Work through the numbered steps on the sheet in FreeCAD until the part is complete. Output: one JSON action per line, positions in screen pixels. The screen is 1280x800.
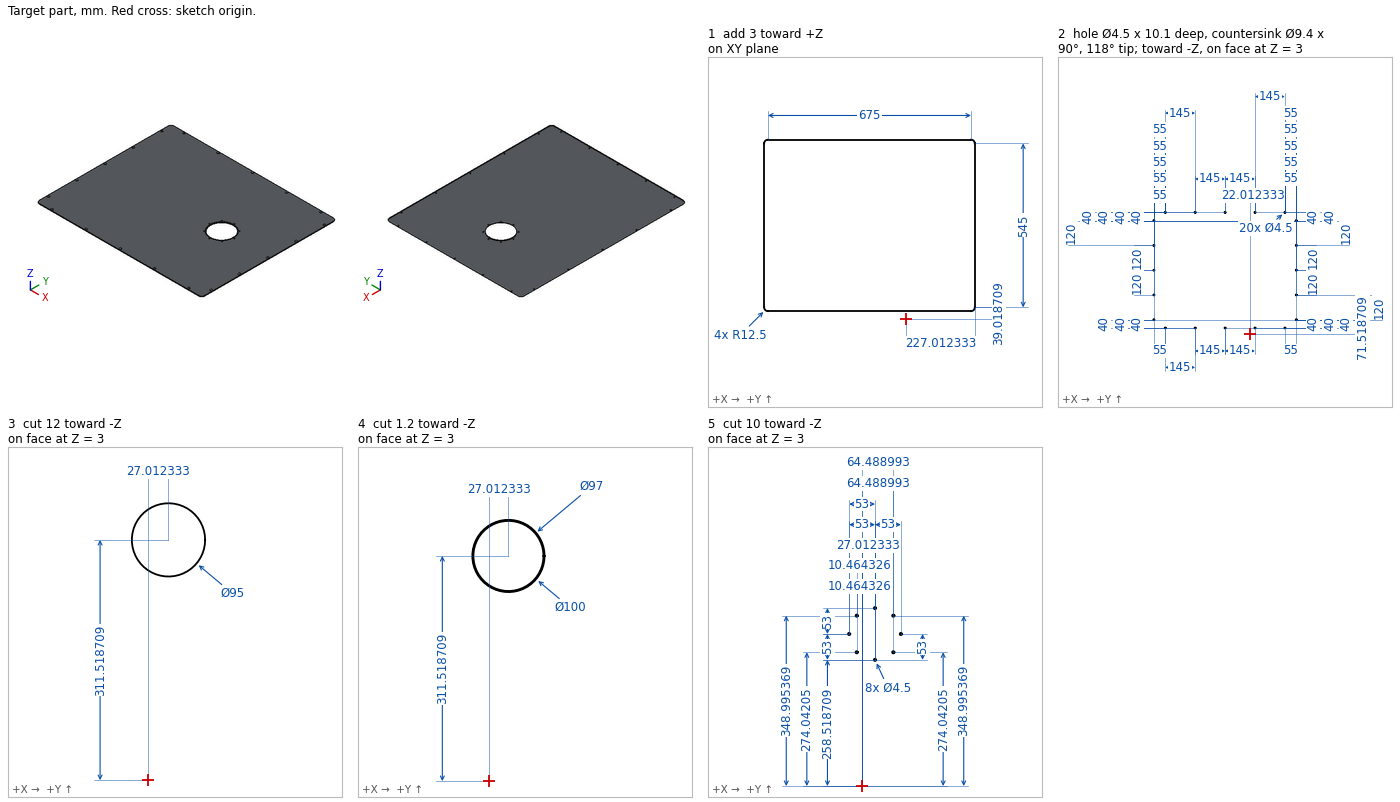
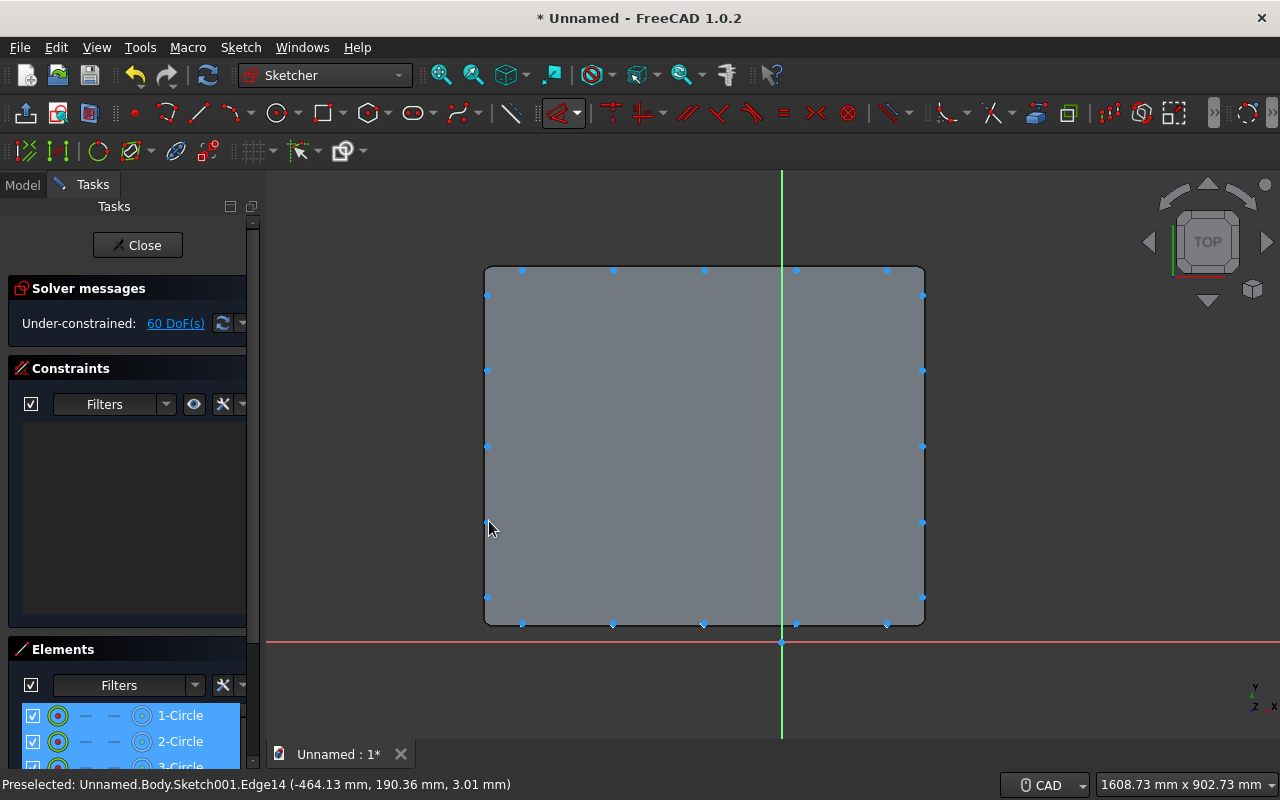
{"action": "scroll", "coordinate": [488, 597], "scroll_direction": "up", "scroll_amount": 11}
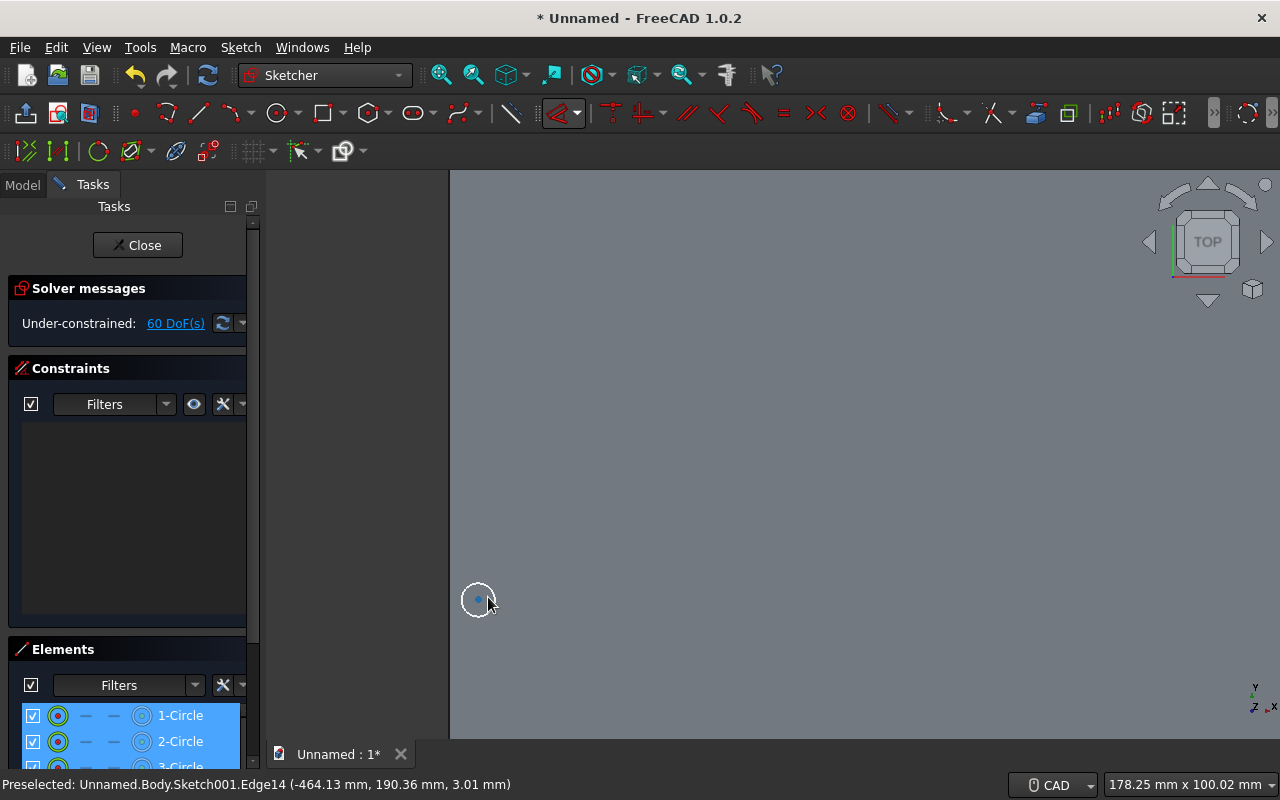
{"action": "left_click", "coordinate": [490, 588]}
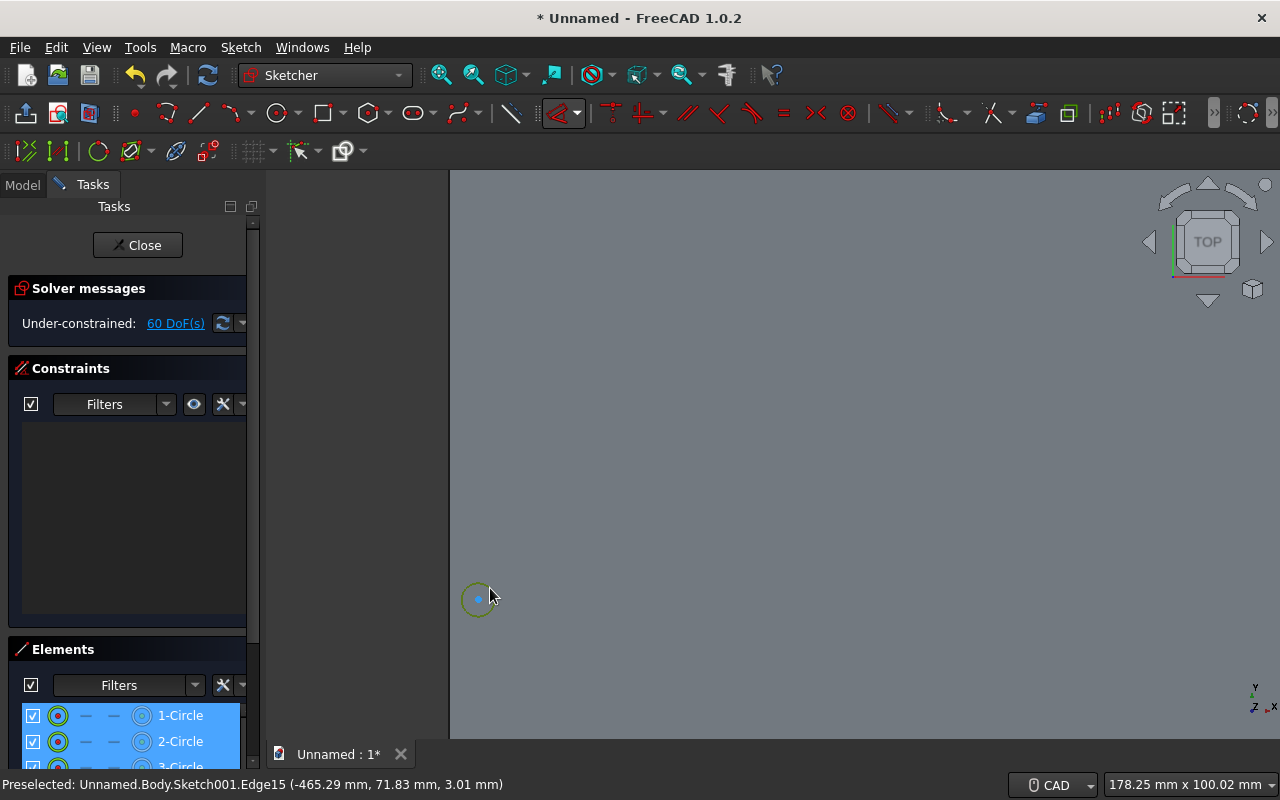
{"action": "scroll", "coordinate": [488, 597], "scroll_direction": "down", "scroll_amount": 11}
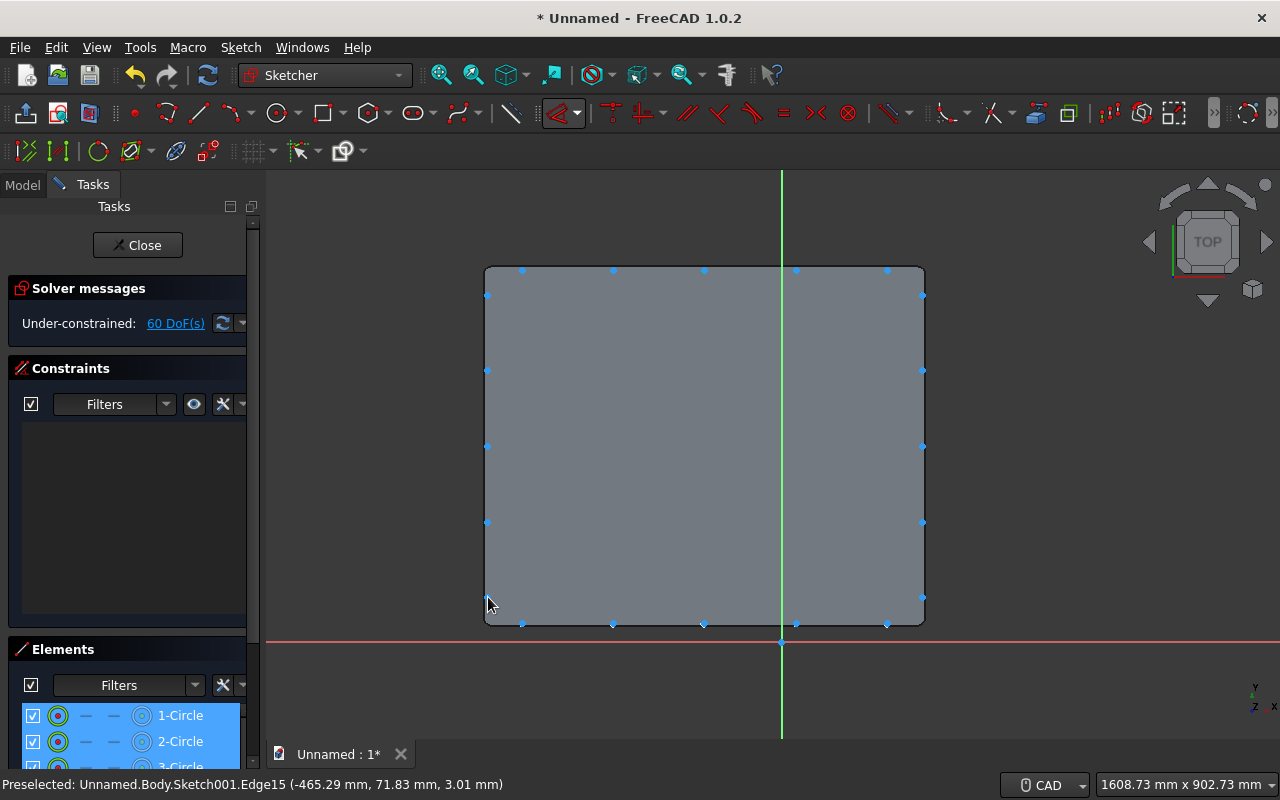
{"action": "scroll", "coordinate": [524, 622], "scroll_direction": "up", "scroll_amount": 9}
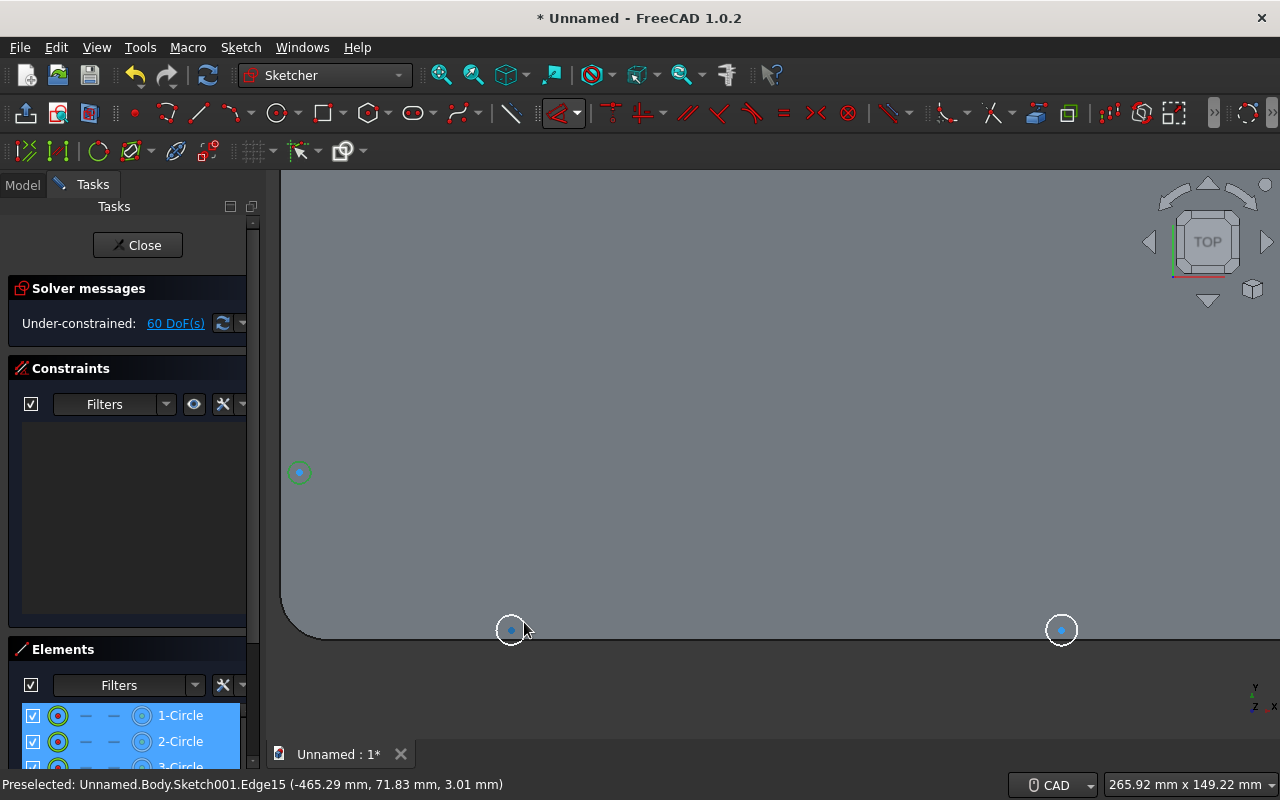
{"action": "left_click", "coordinate": [522, 620]}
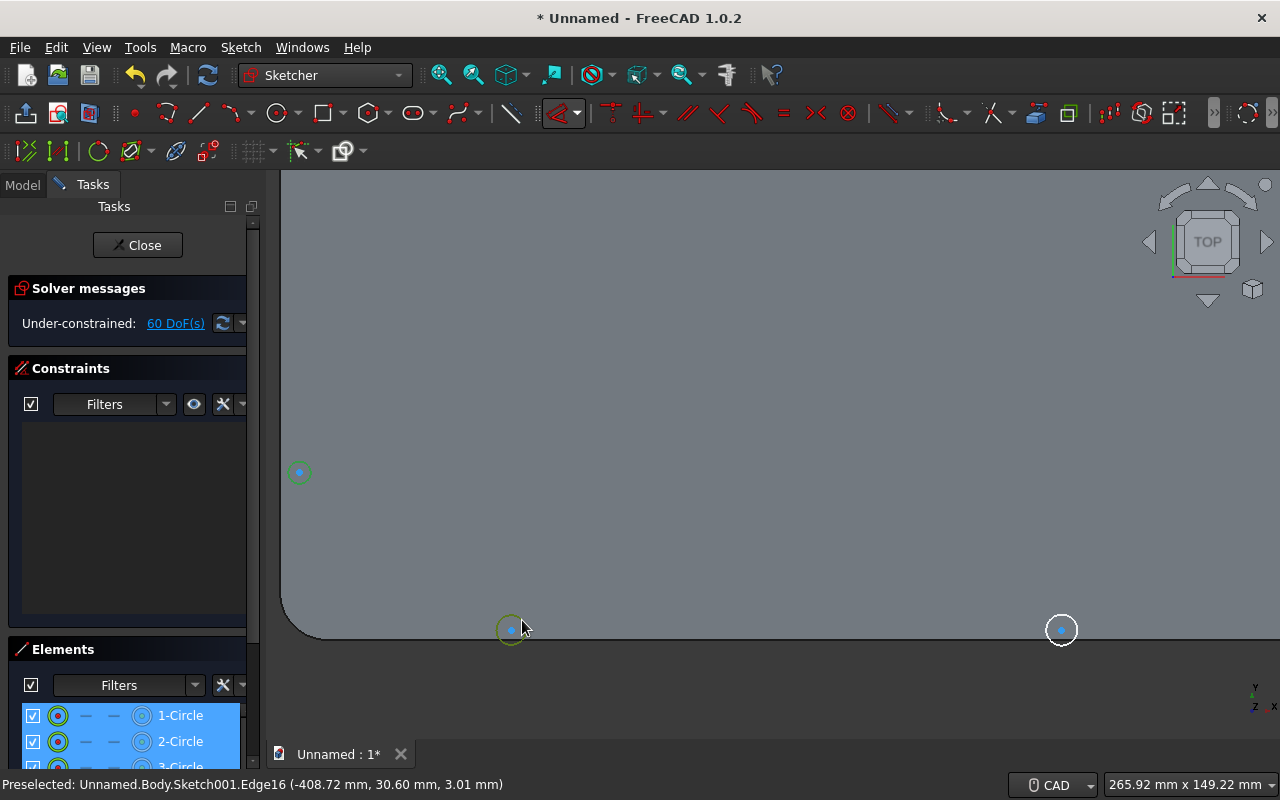
{"action": "left_click", "coordinate": [1073, 619]}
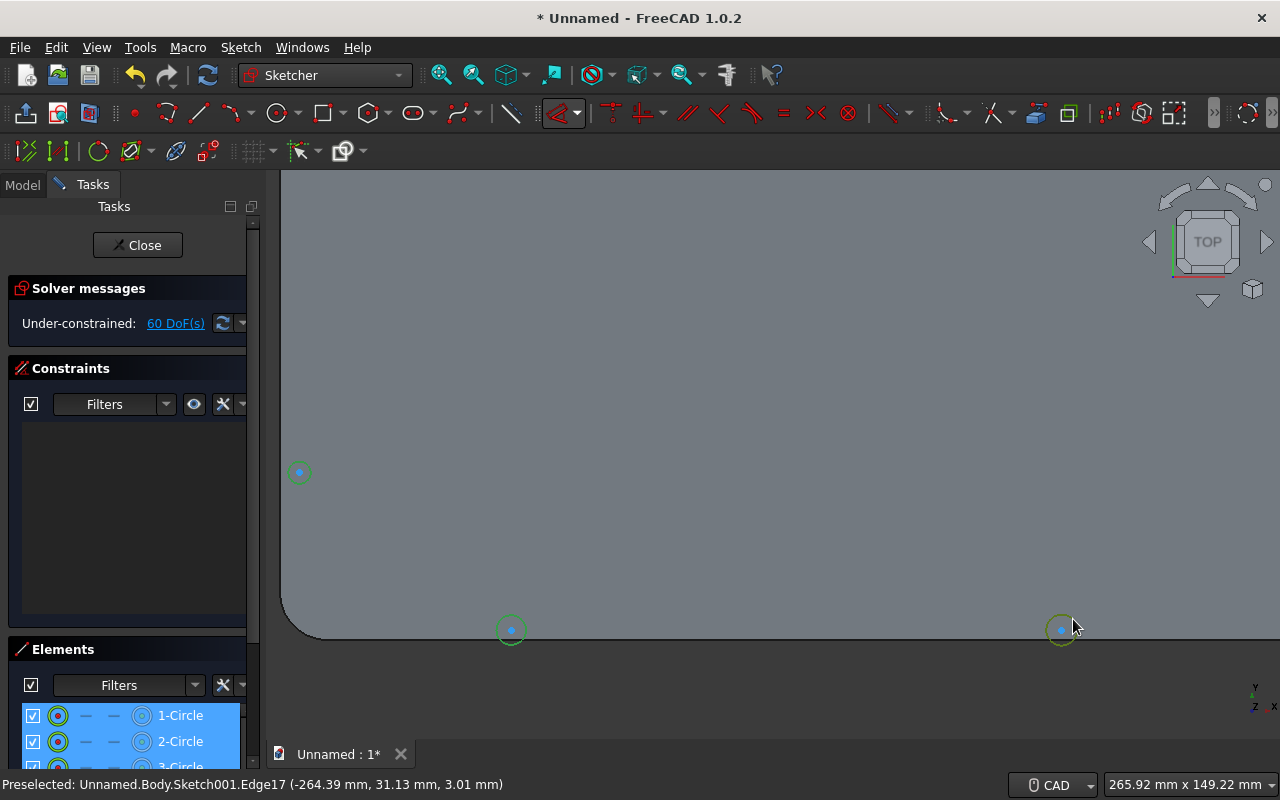
{"action": "scroll", "coordinate": [524, 622], "scroll_direction": "down", "scroll_amount": 9}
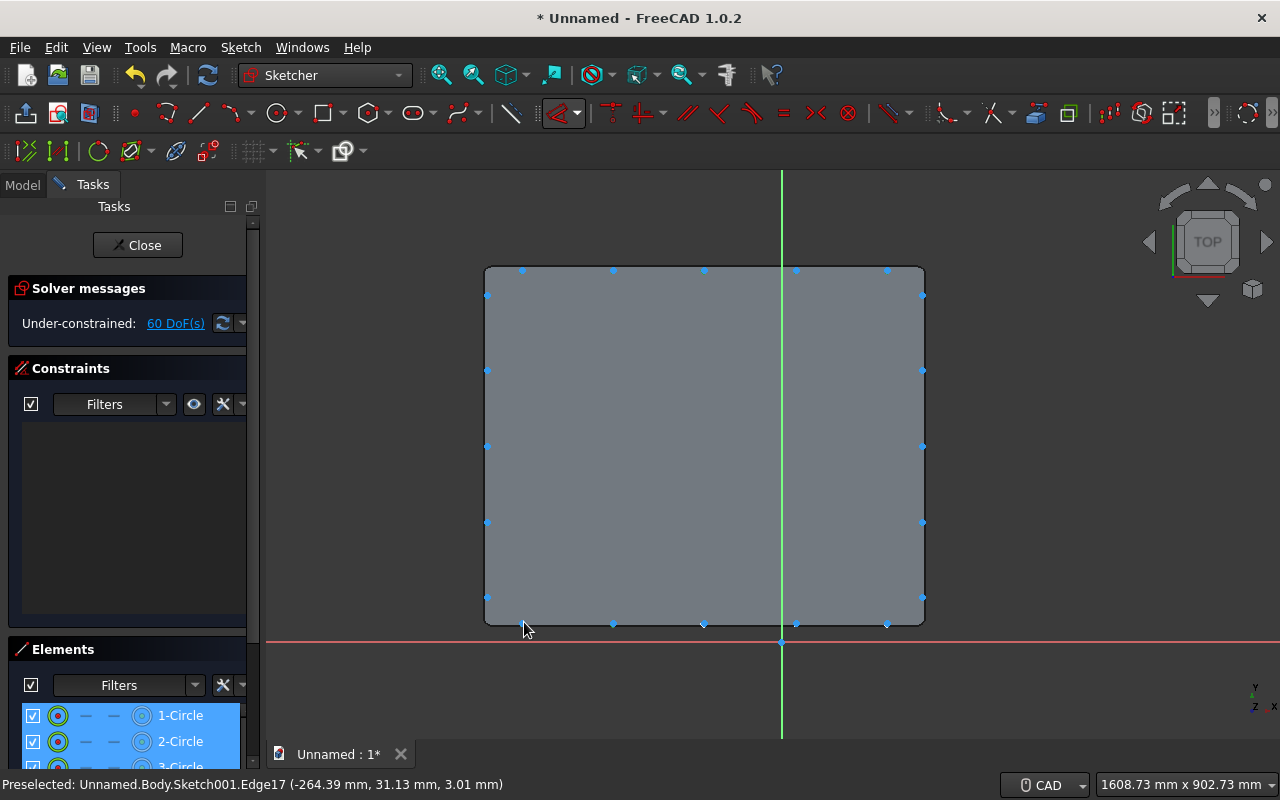
{"action": "scroll", "coordinate": [706, 622], "scroll_direction": "up", "scroll_amount": 9}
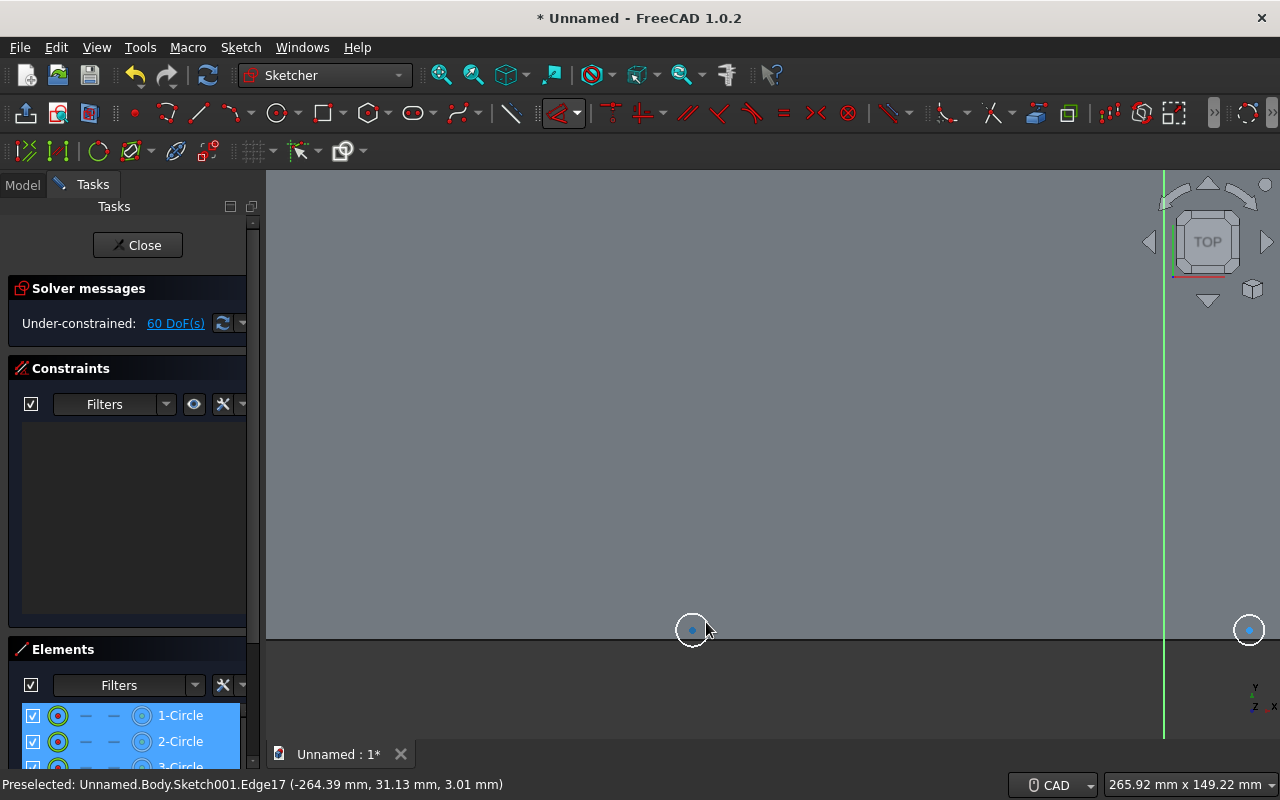
{"action": "left_click", "coordinate": [704, 618]}